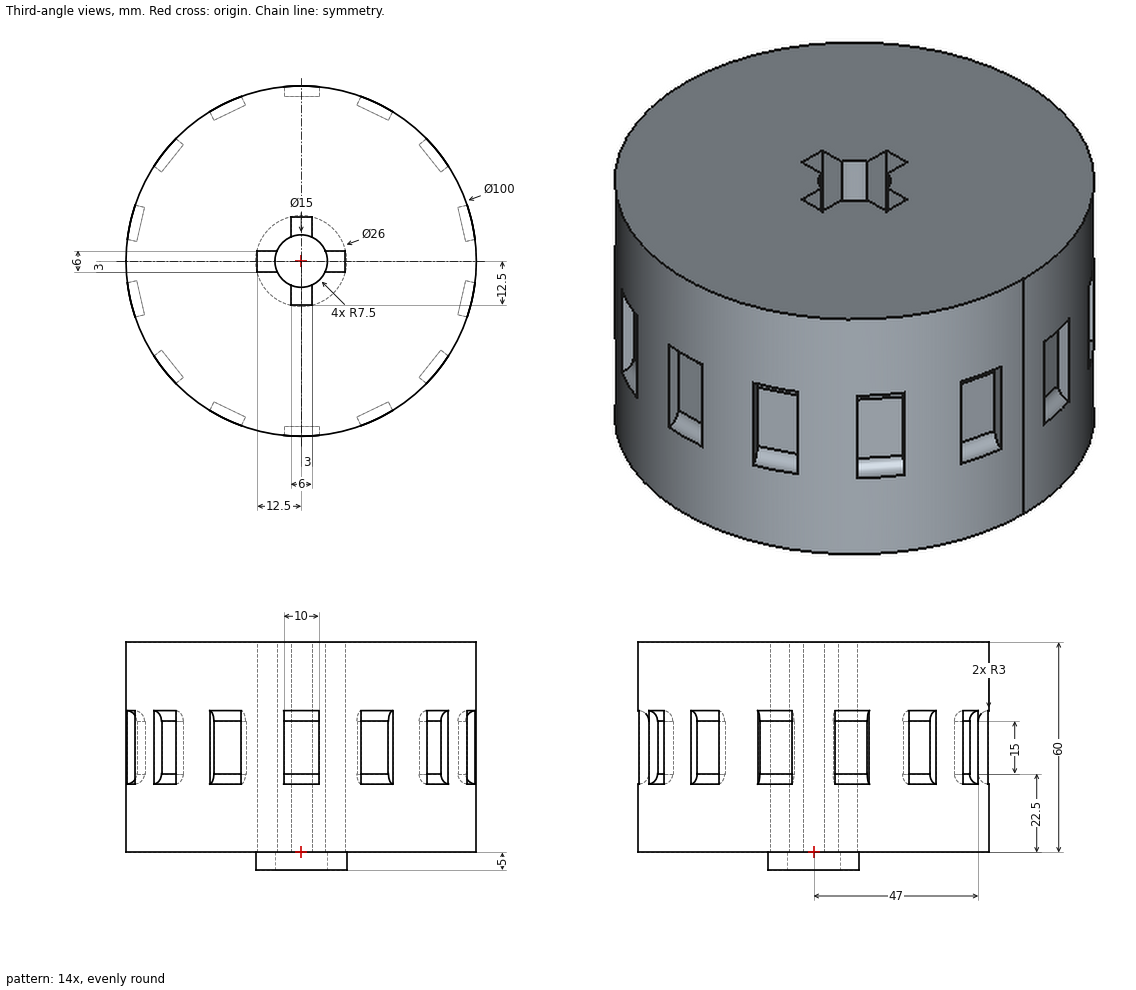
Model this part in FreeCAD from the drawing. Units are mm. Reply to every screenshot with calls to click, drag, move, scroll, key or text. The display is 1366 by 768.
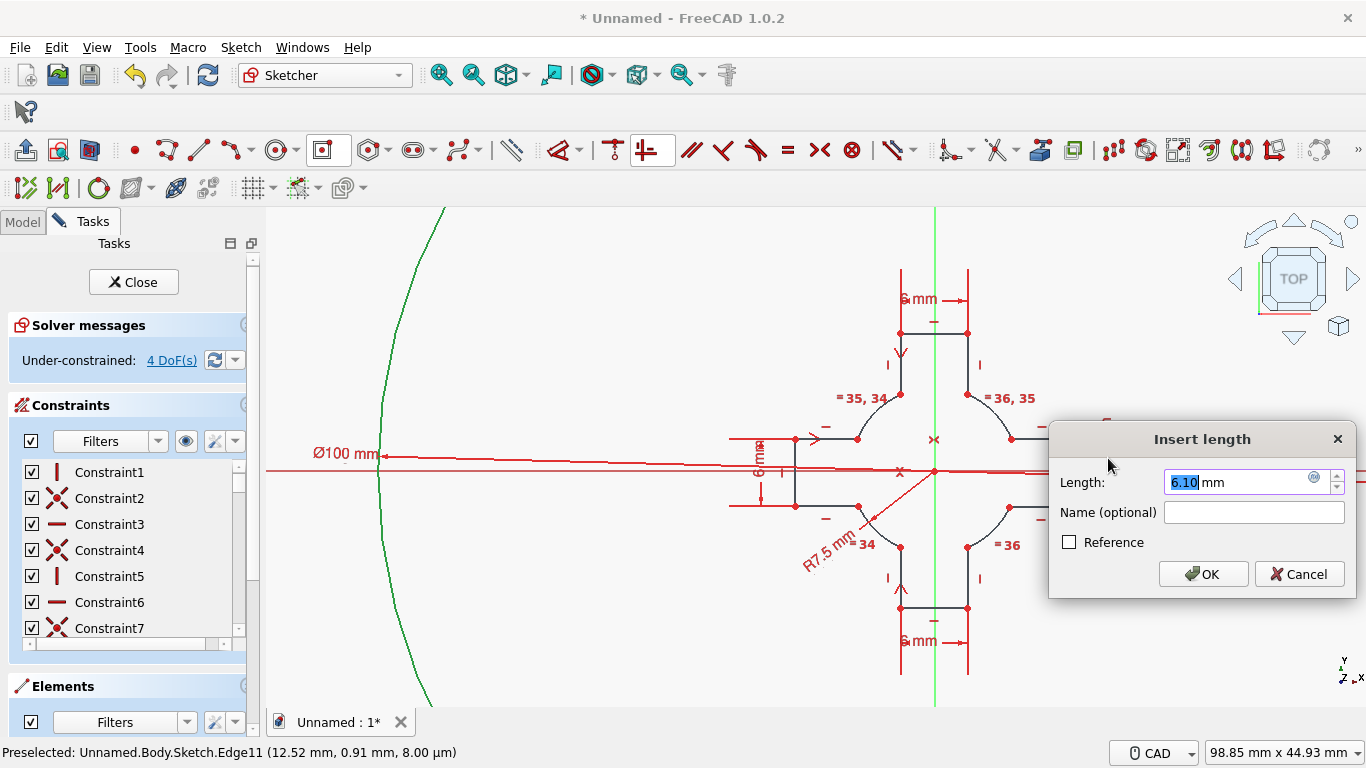
text(6)
key(Return)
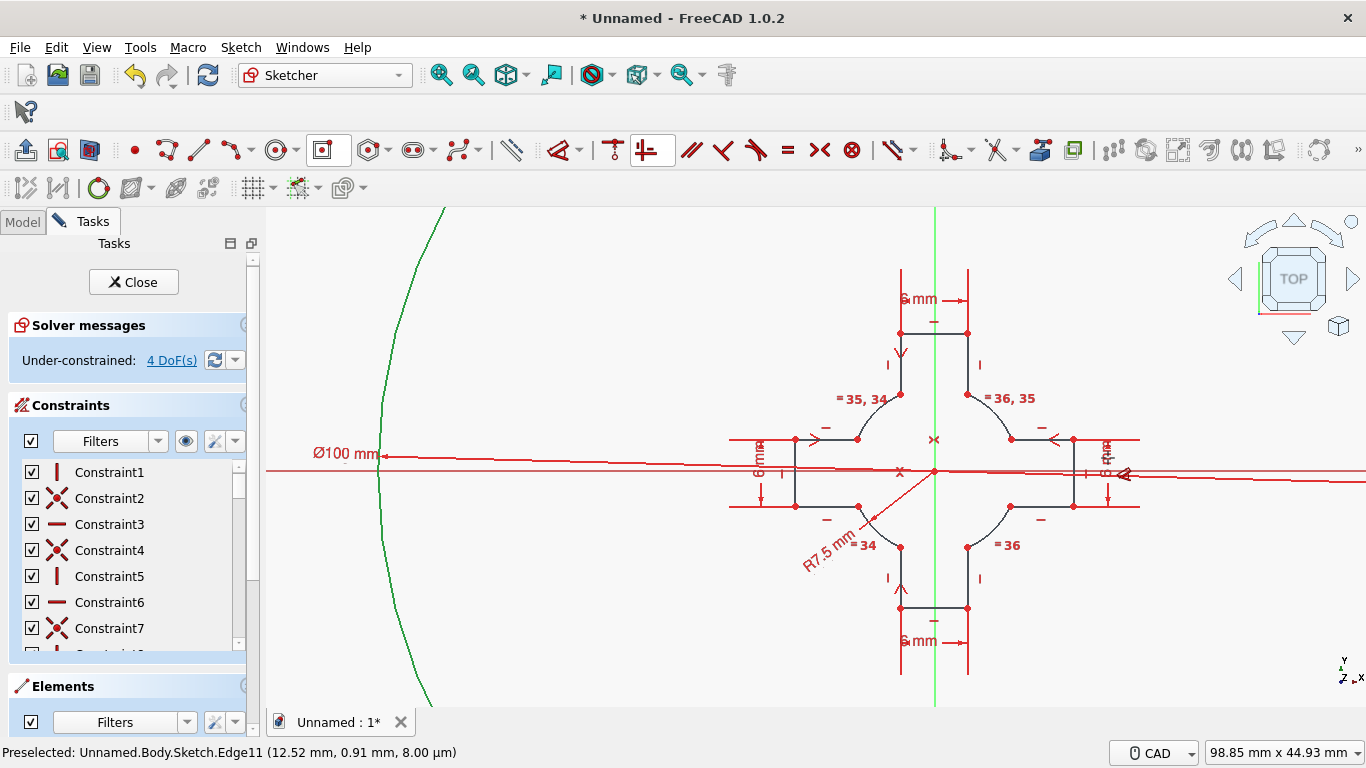
click(968, 548)
click(951, 582)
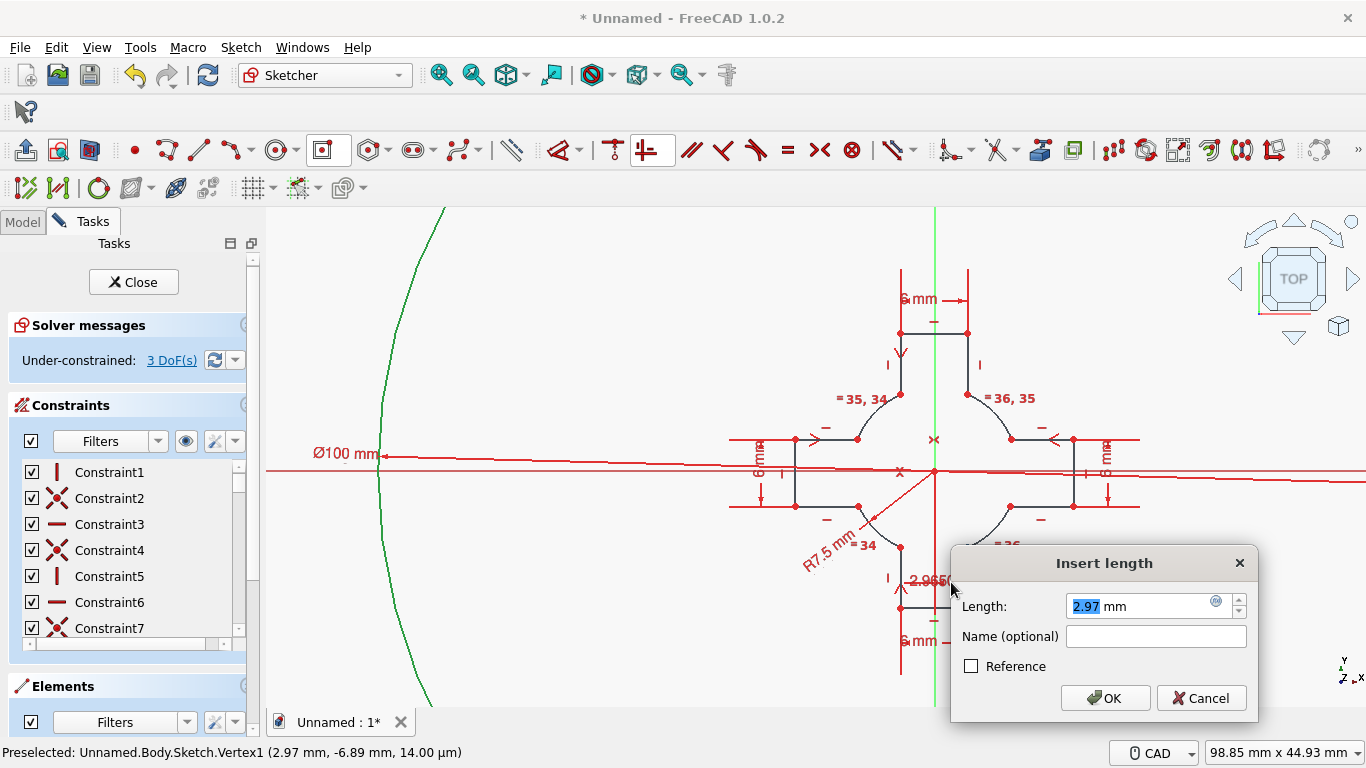
text(3)
key(Return)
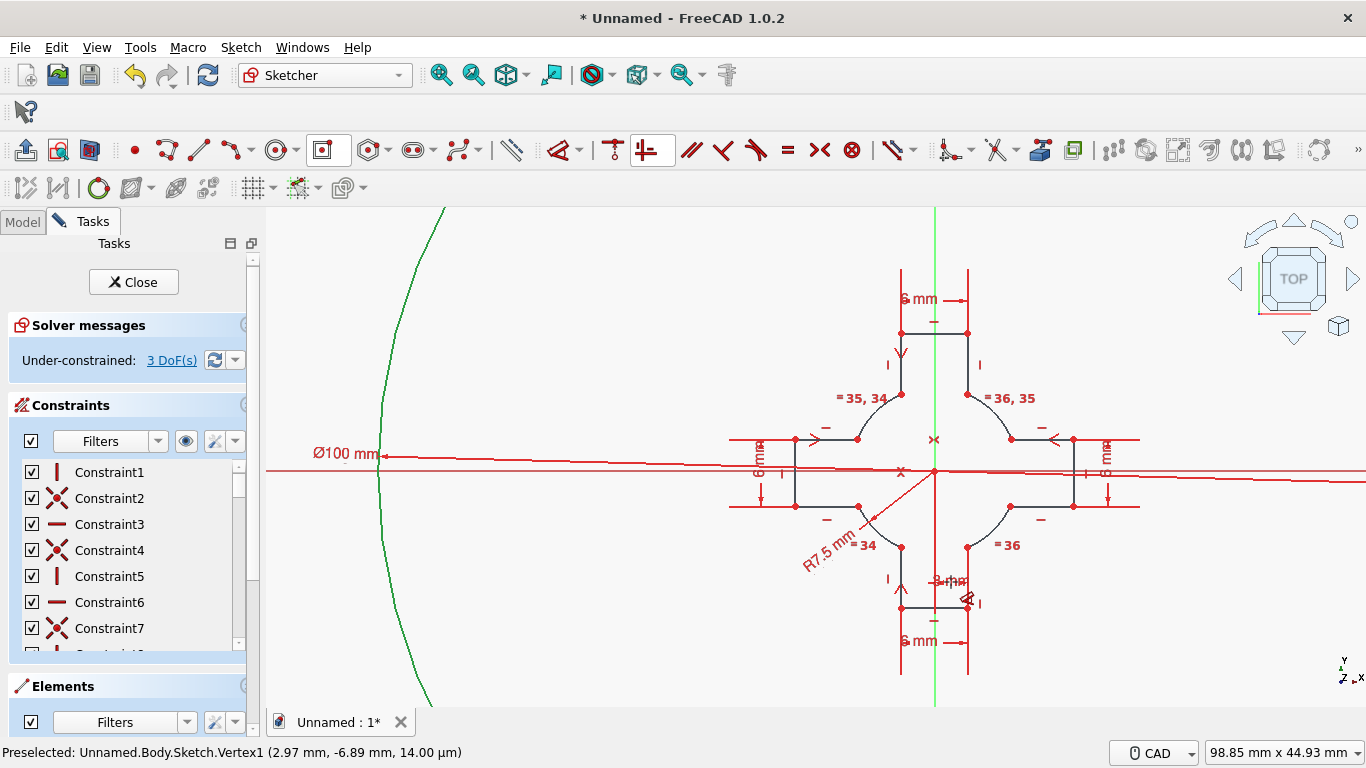
click(859, 507)
click(825, 489)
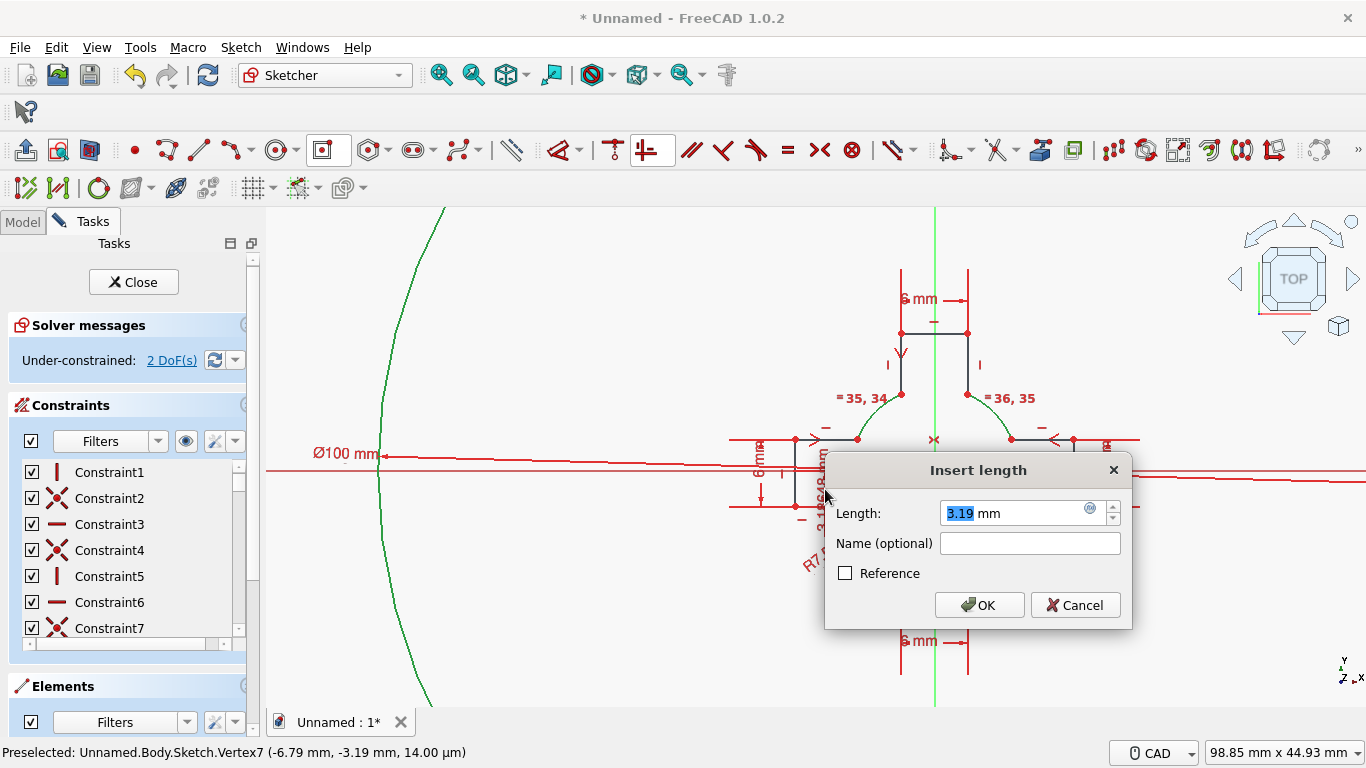
text(3)
key(Return)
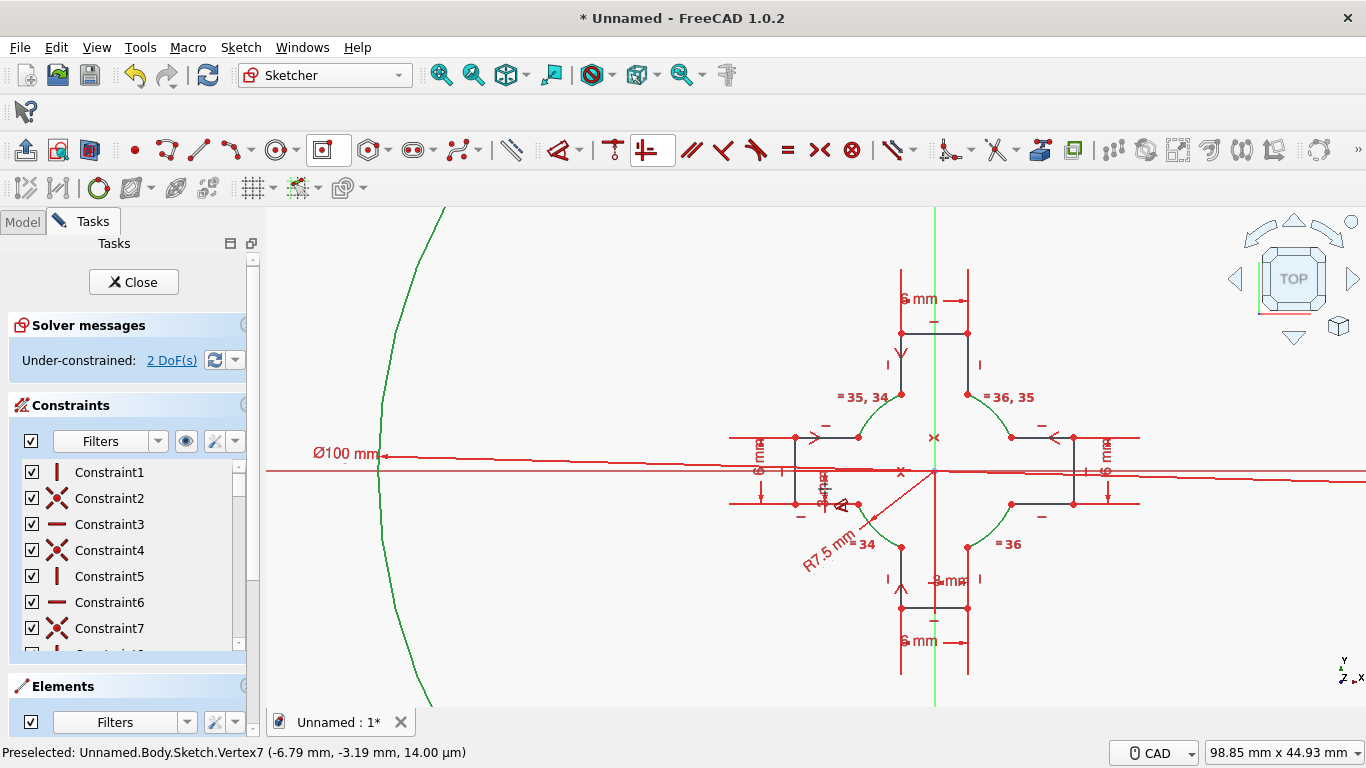
click(968, 608)
click(1002, 492)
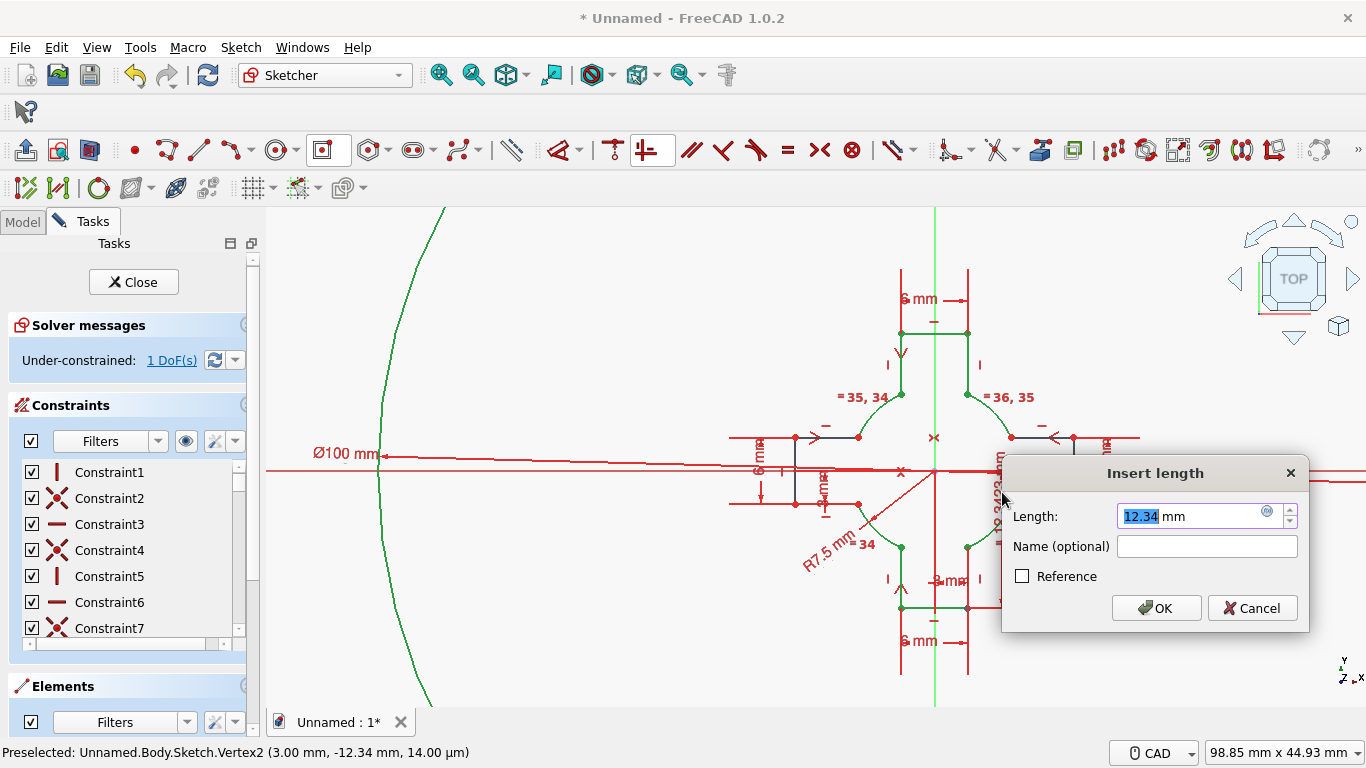
text(12.5)
key(Return)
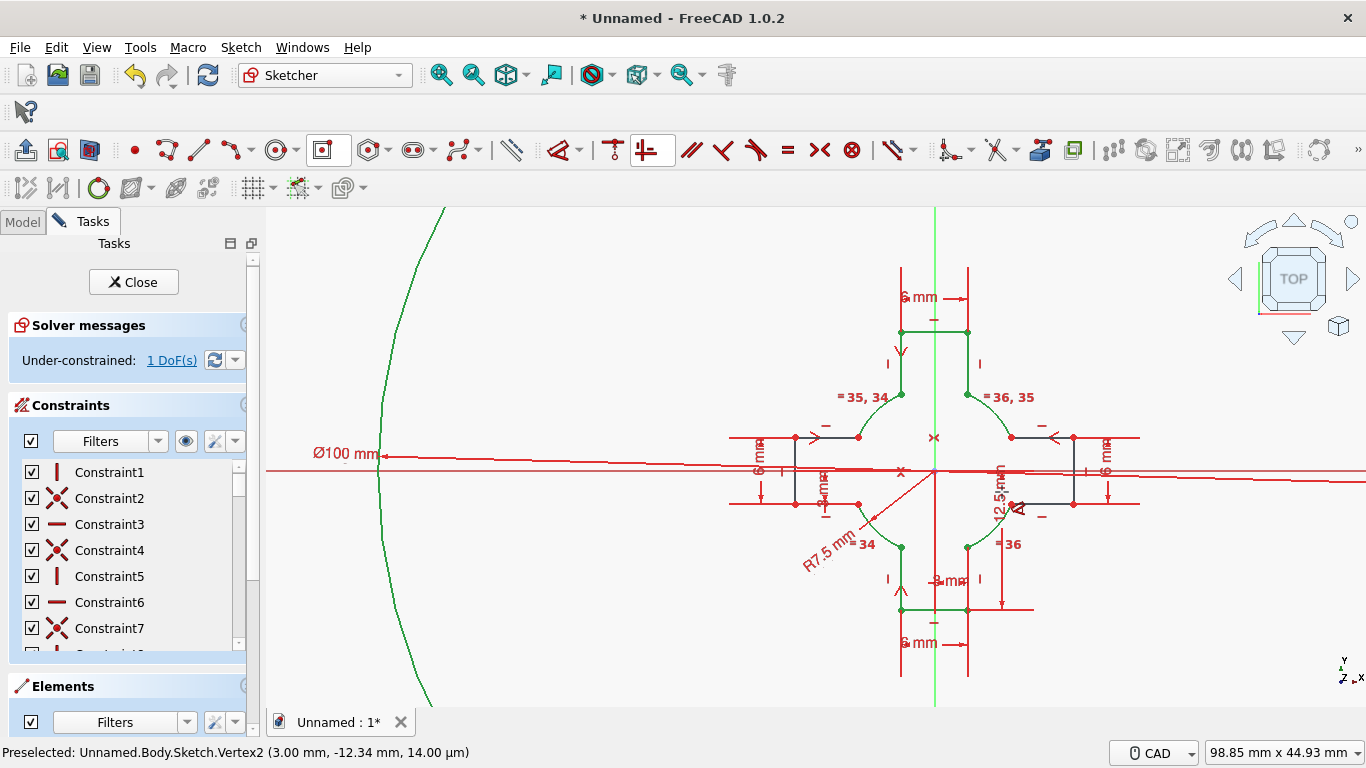
click(795, 504)
click(914, 538)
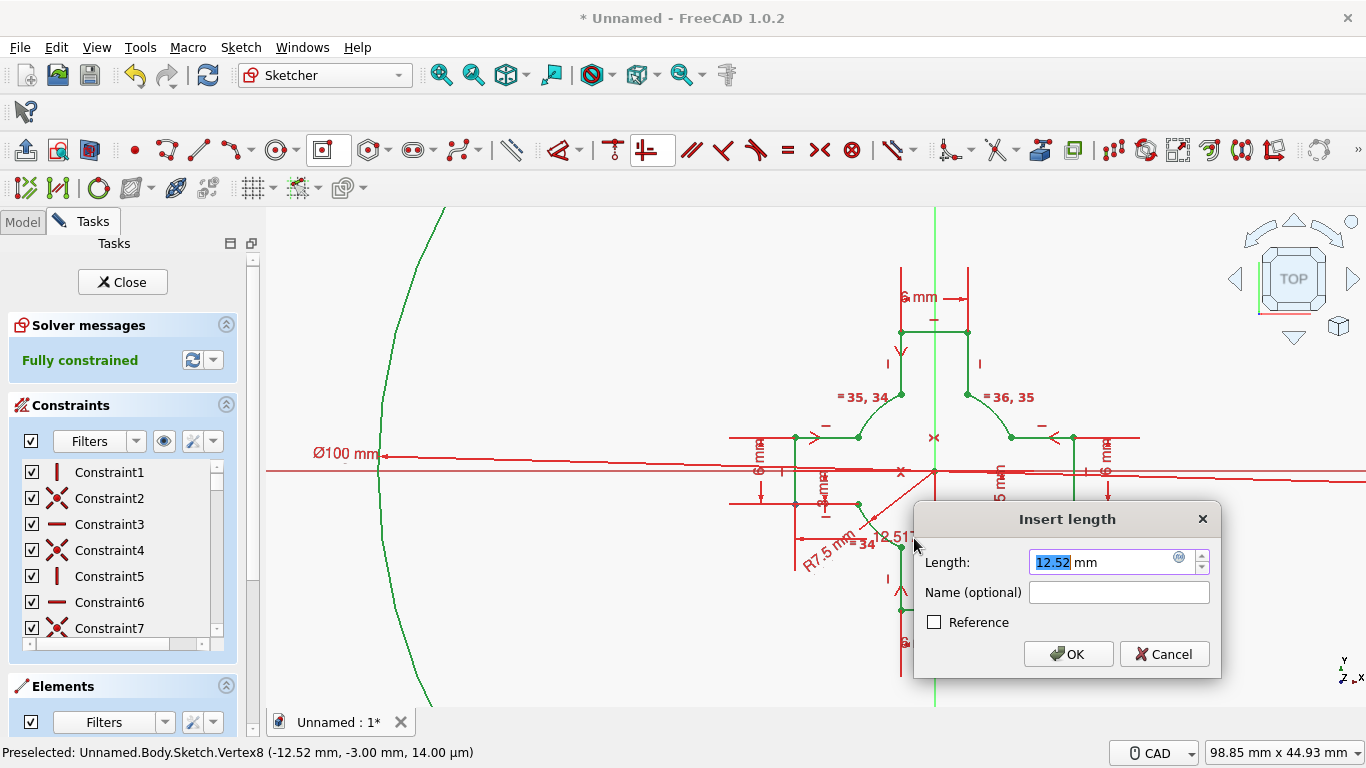
text(12.5)
key(Return)
key(Escape)